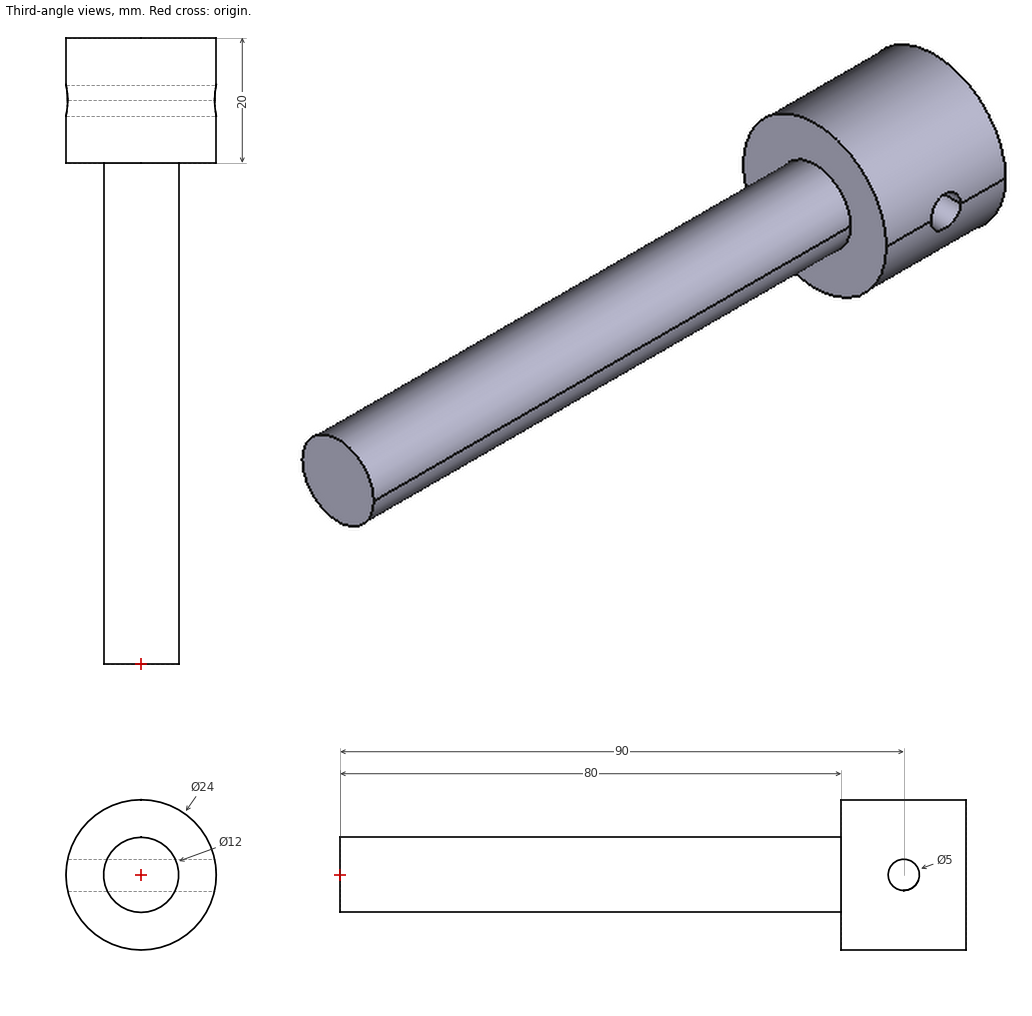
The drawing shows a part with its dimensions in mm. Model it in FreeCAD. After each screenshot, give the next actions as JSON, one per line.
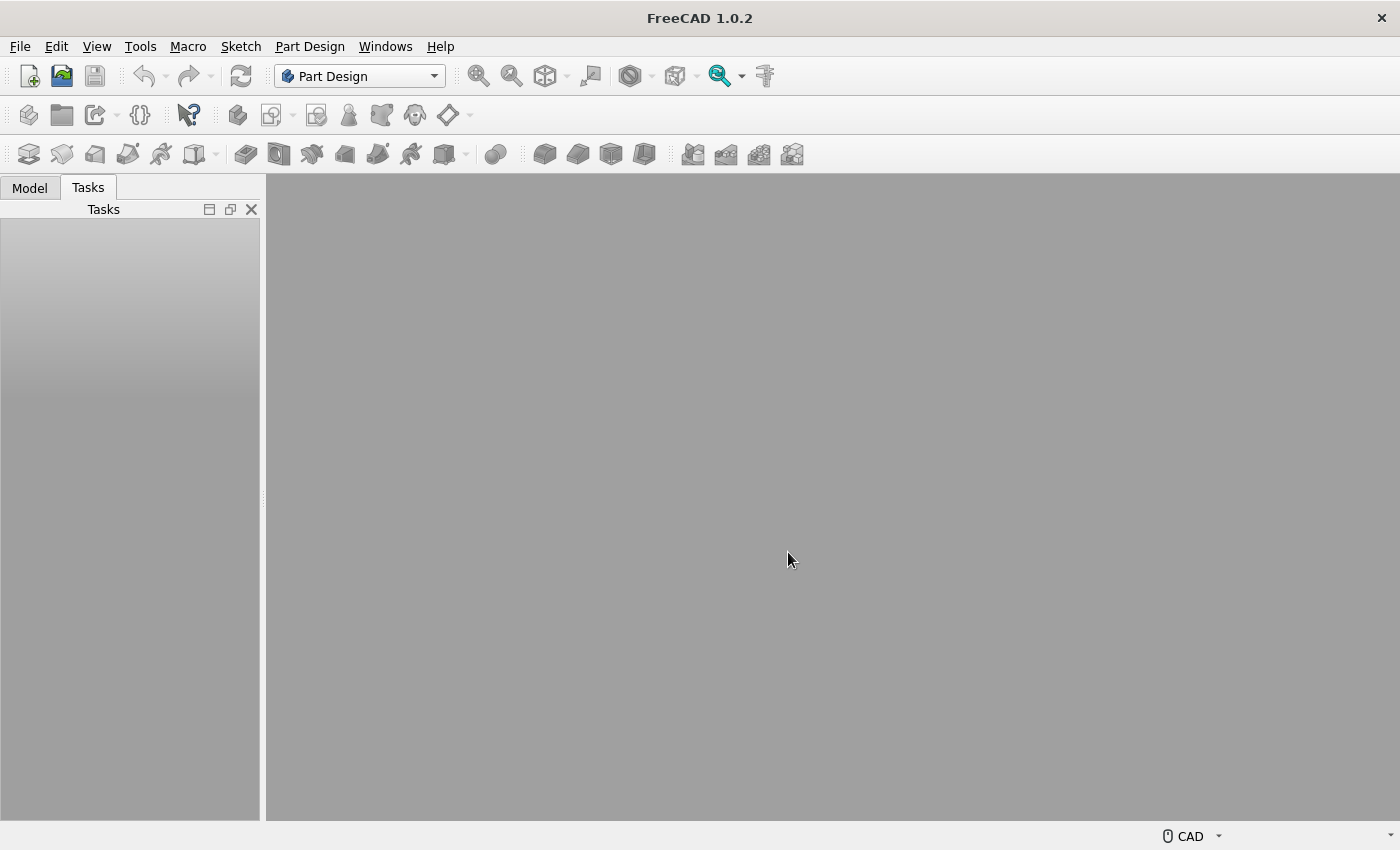
{"action": "left_click", "coordinate": [29, 76]}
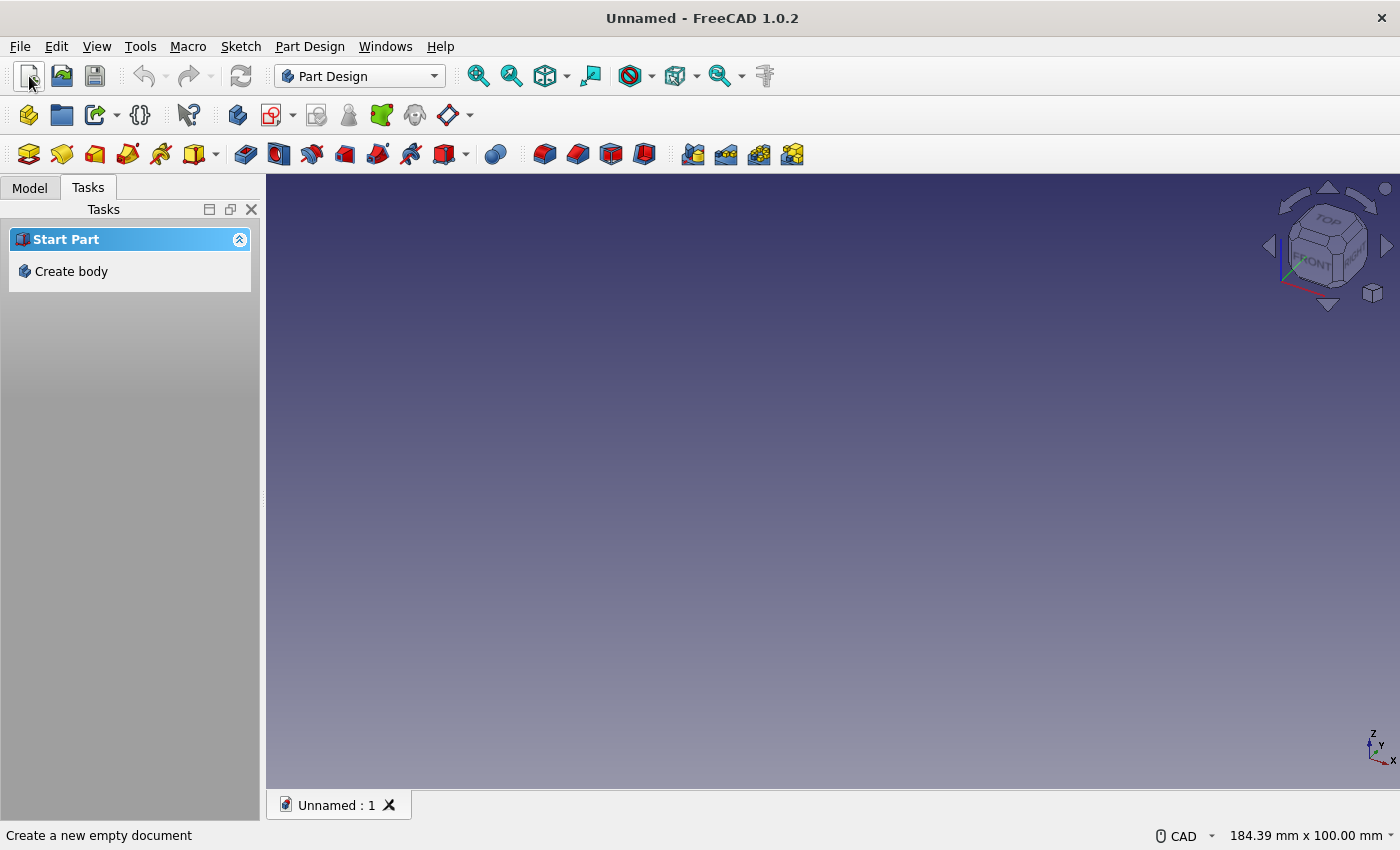
{"action": "left_click", "coordinate": [270, 116]}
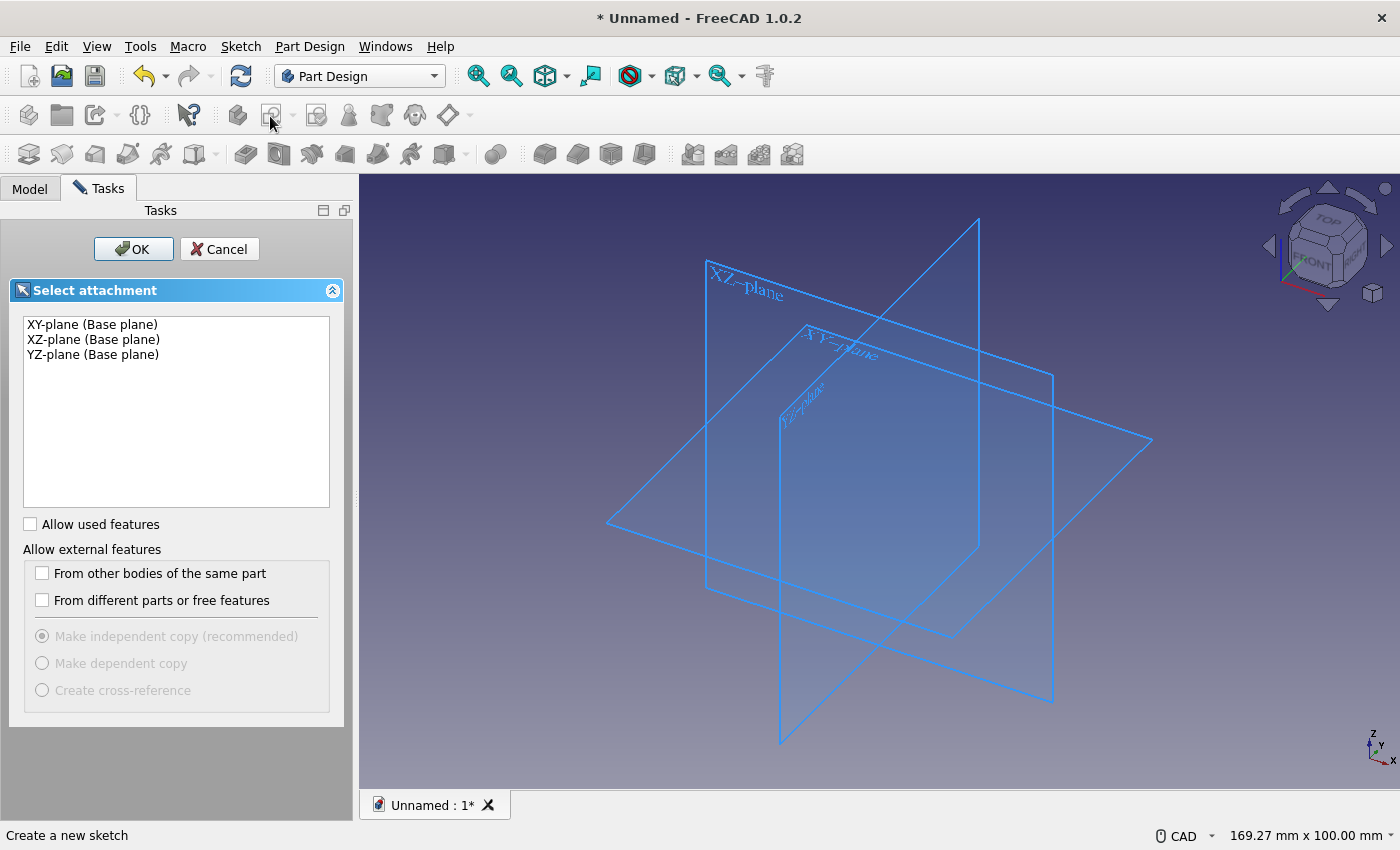
{"action": "left_click", "coordinate": [84, 340]}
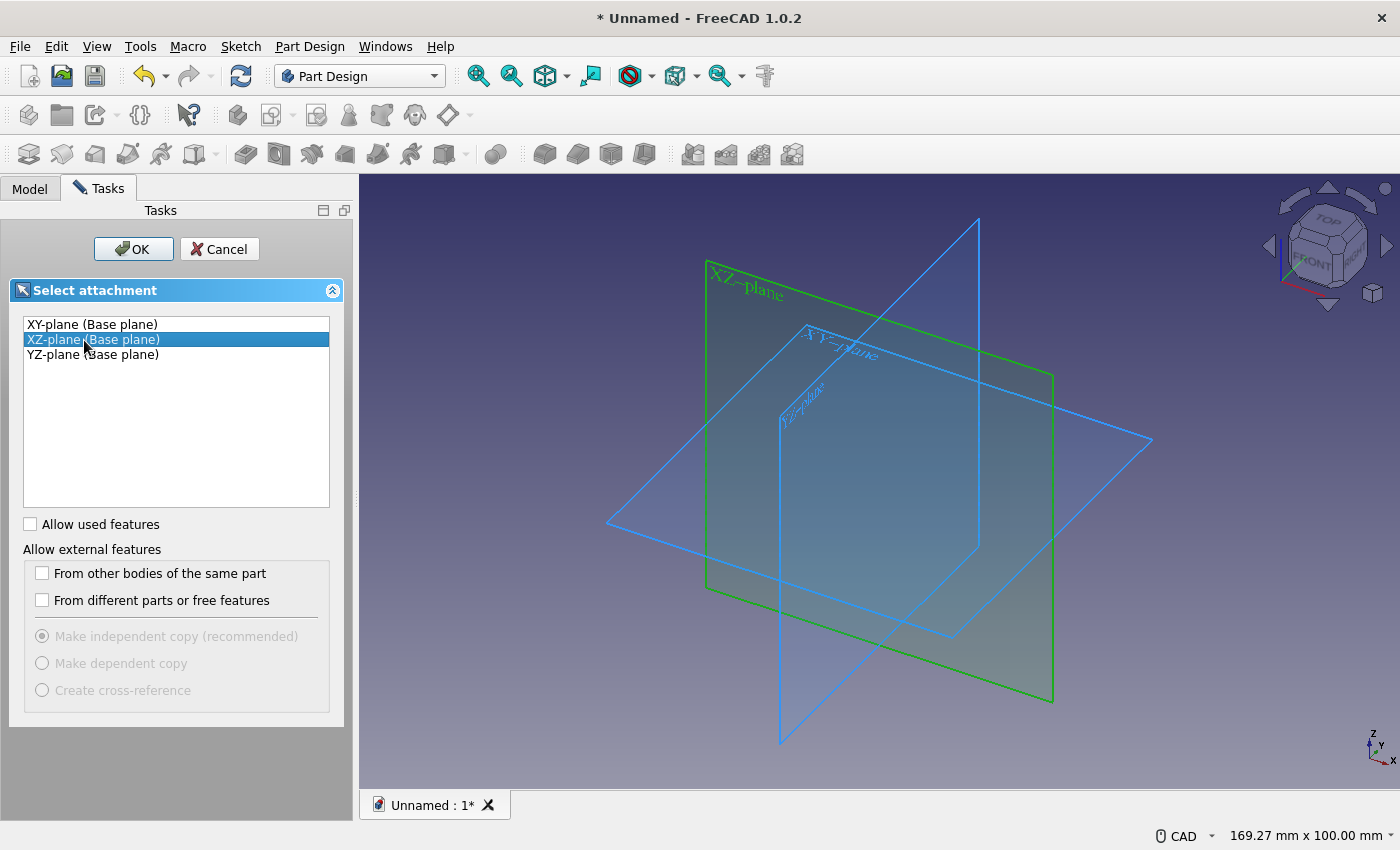
{"action": "left_click", "coordinate": [134, 249]}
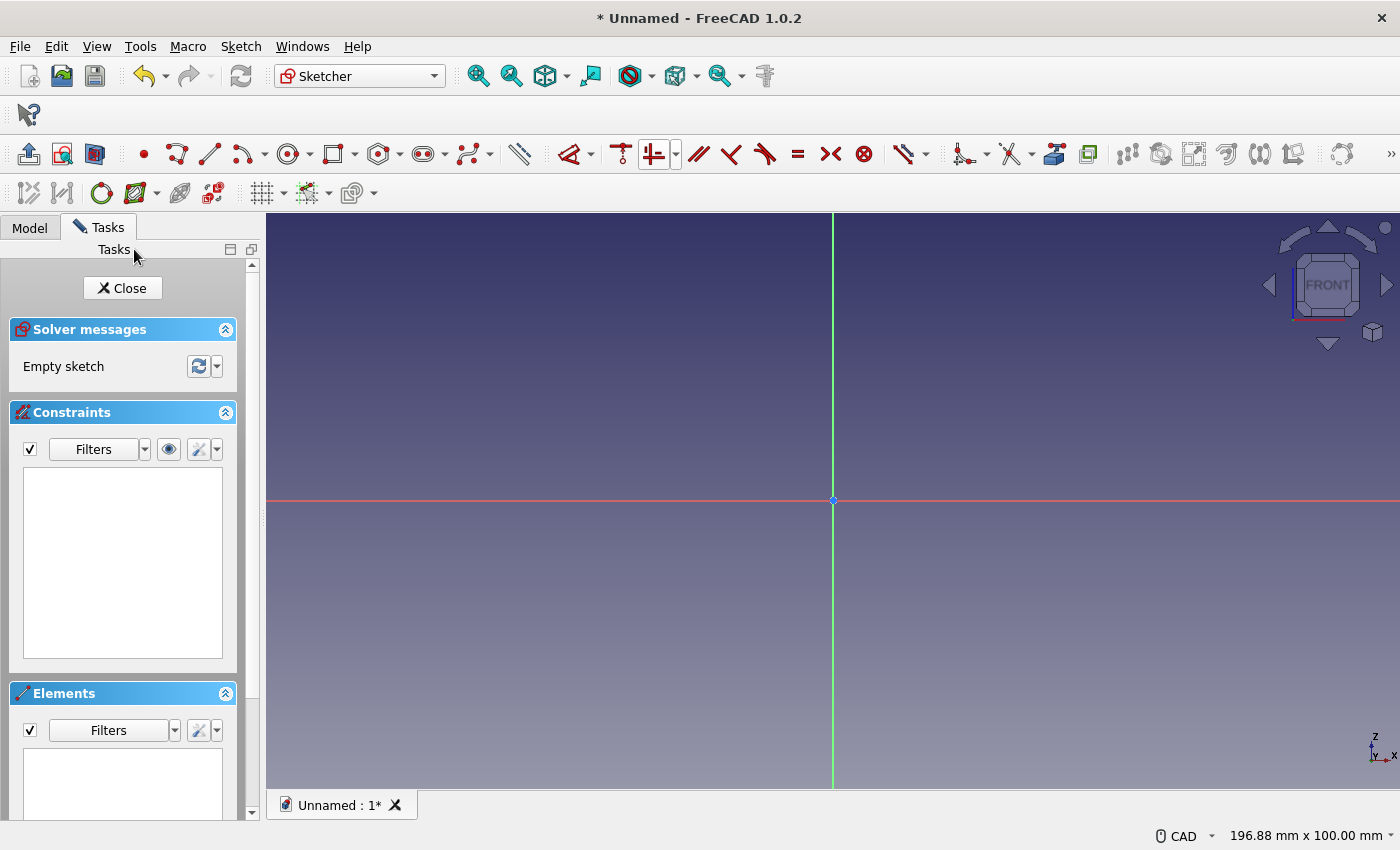
{"action": "scroll", "coordinate": [850, 501], "scroll_direction": "up", "scroll_amount": 8}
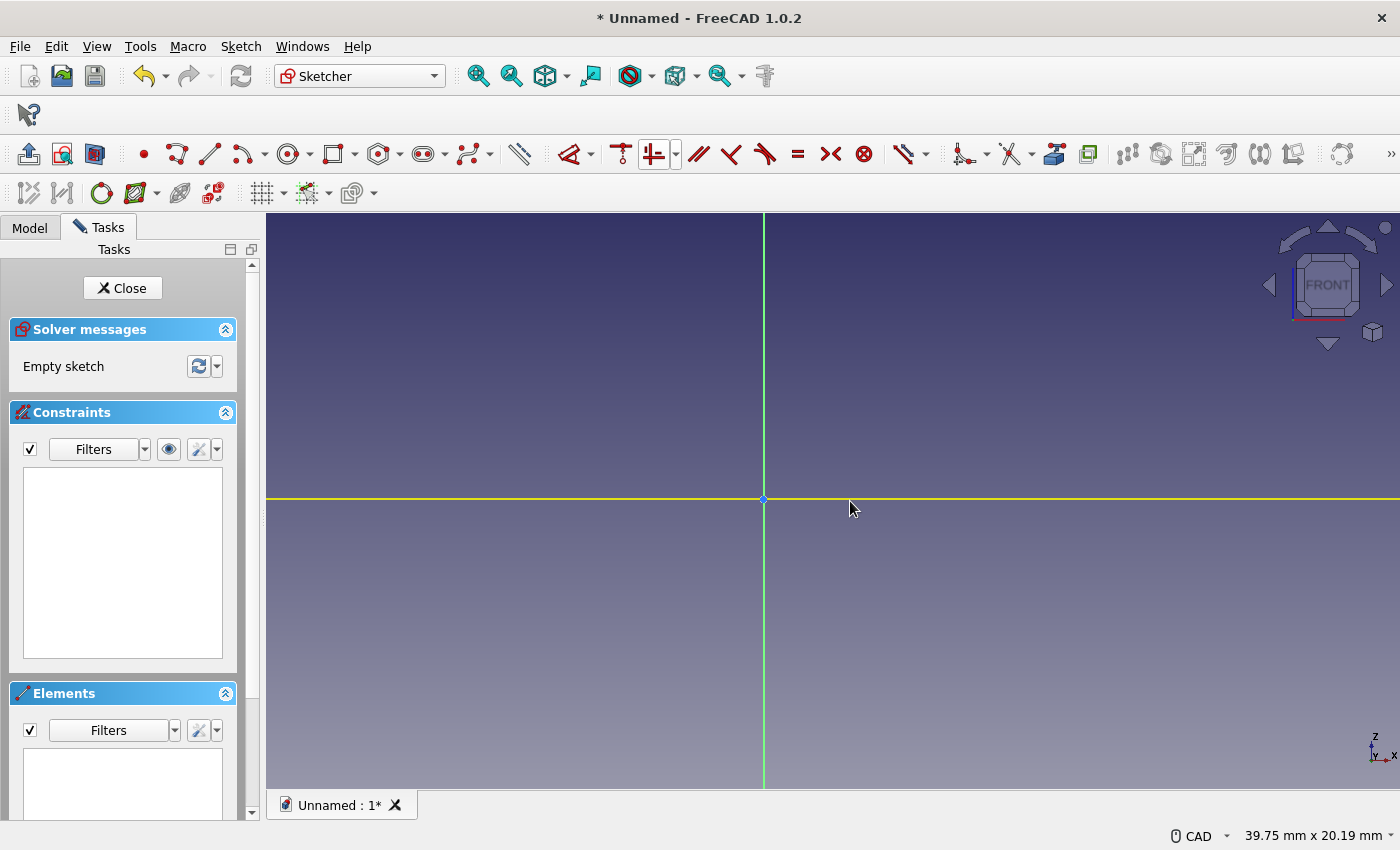
{"action": "left_click", "coordinate": [288, 154]}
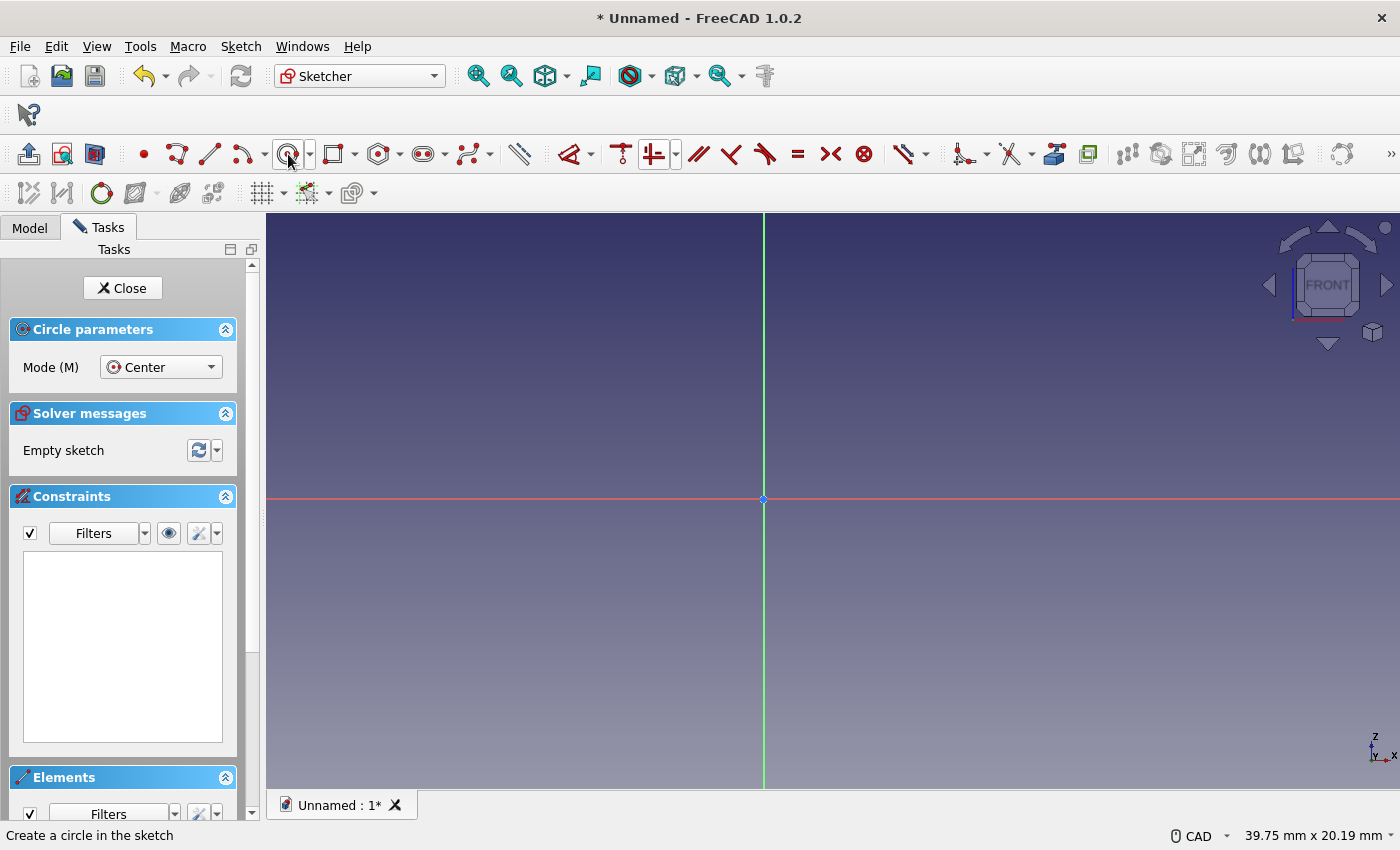
{"action": "left_click", "coordinate": [764, 499]}
{"action": "left_click", "coordinate": [885, 378]}
{"action": "key", "text": "Escape"}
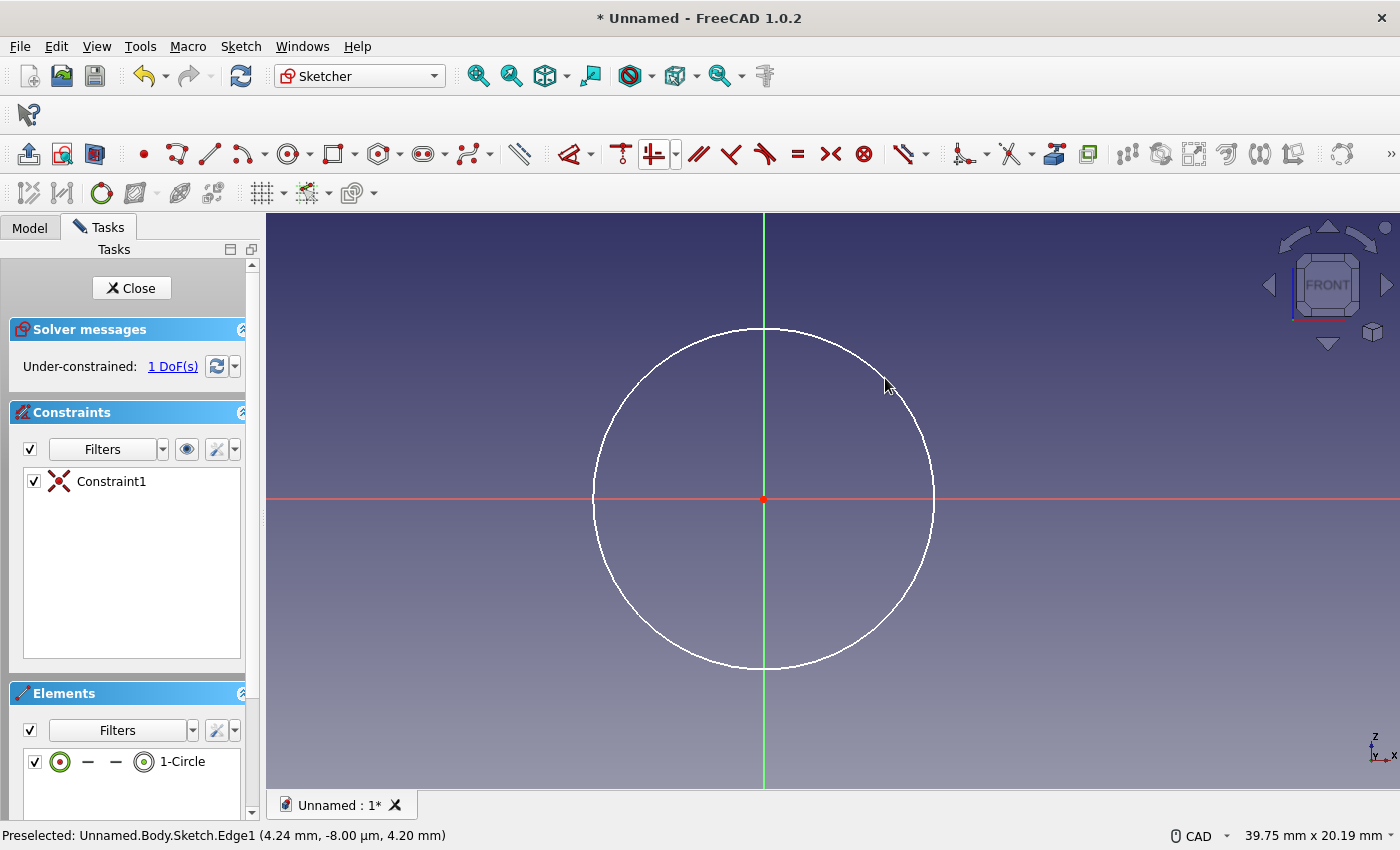
{"action": "left_click", "coordinate": [884, 378]}